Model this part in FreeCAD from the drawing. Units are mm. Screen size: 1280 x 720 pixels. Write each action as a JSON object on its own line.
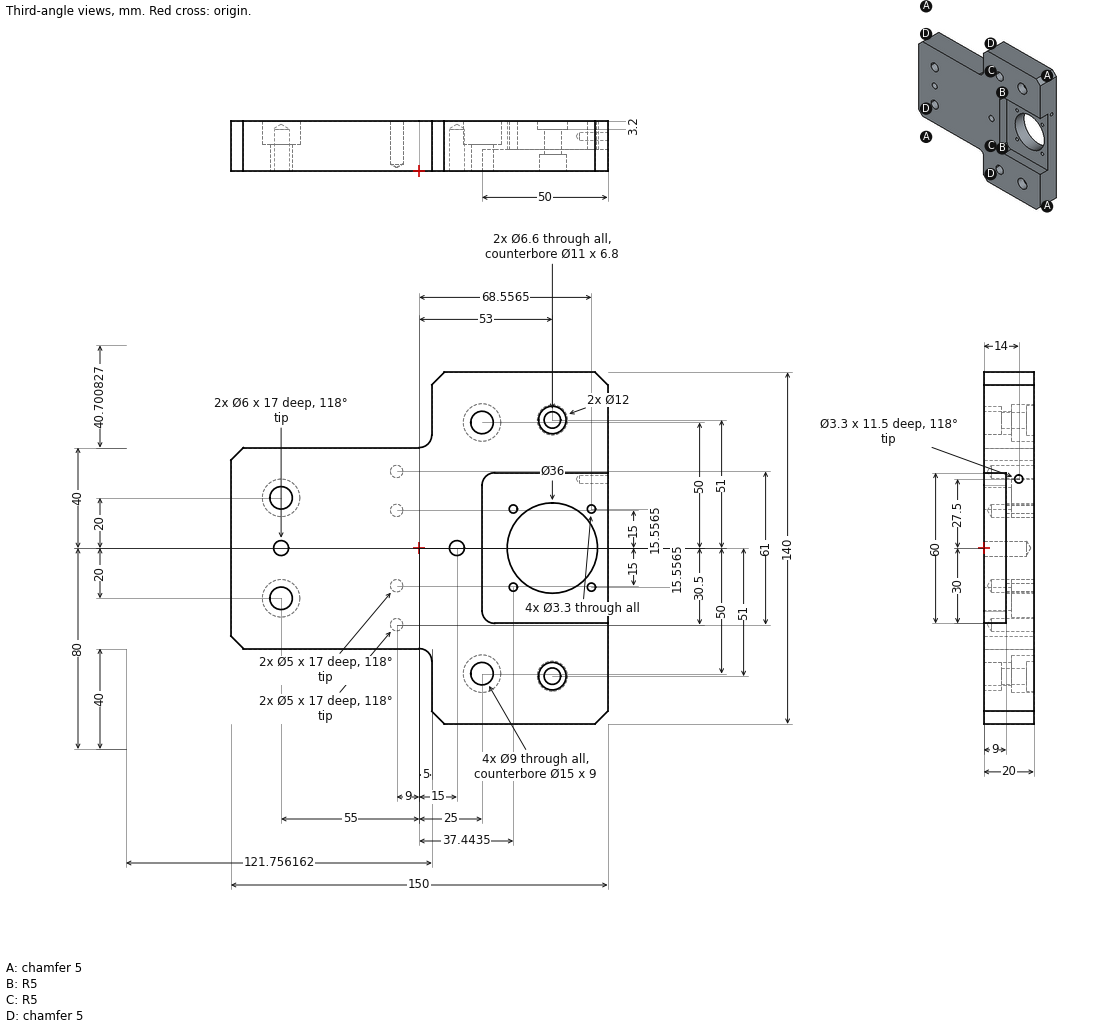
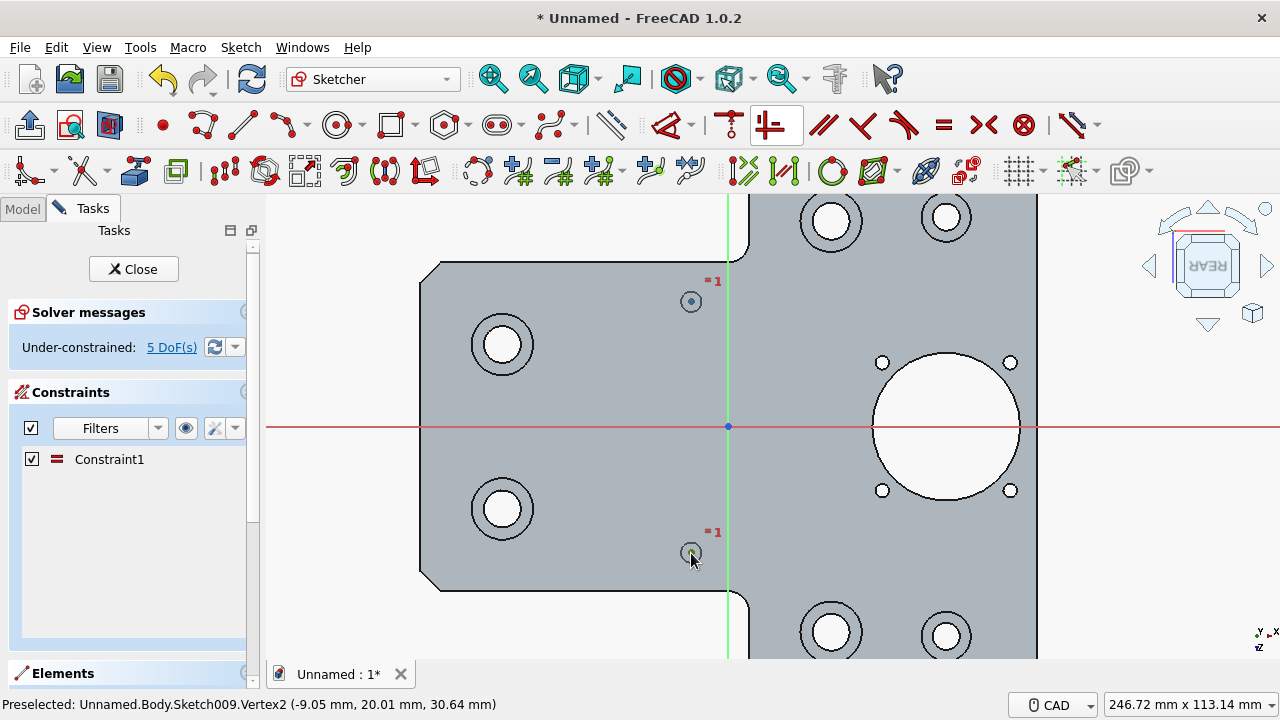
{"action": "key", "text": "v"}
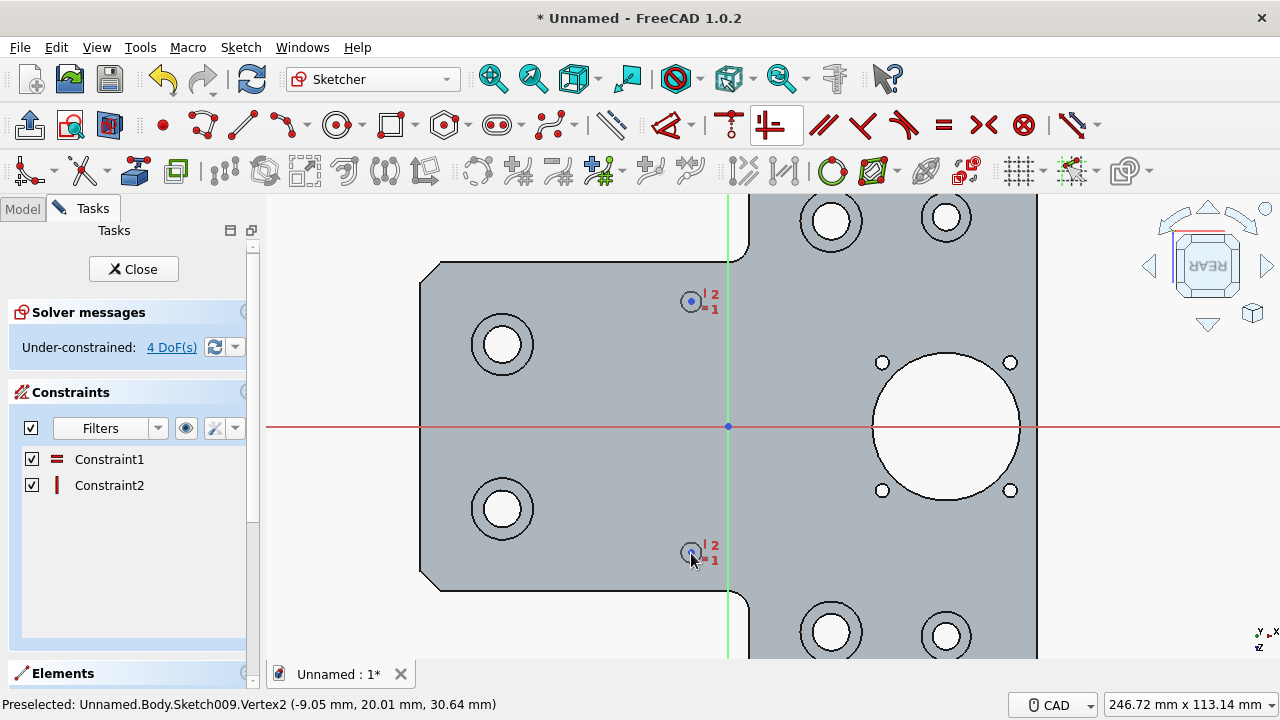
{"action": "left_click", "coordinate": [666, 126]}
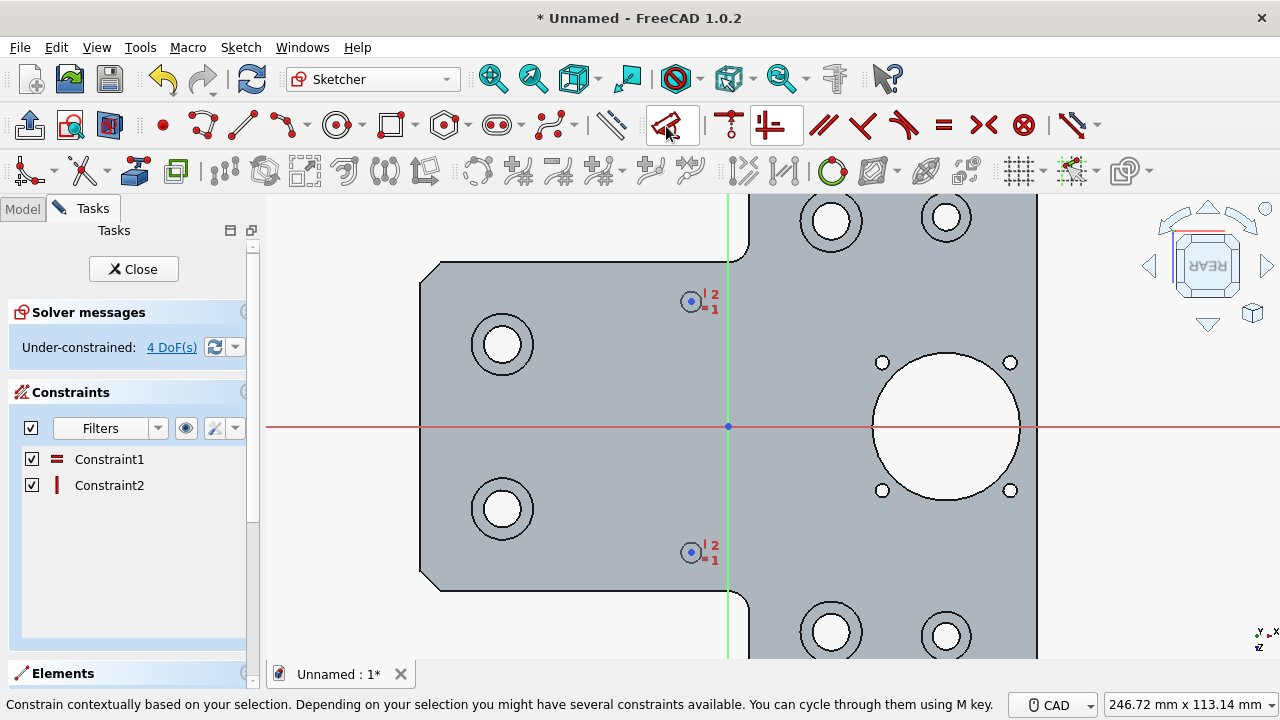
{"action": "scroll", "coordinate": [698, 295], "scroll_direction": "up", "scroll_amount": 4}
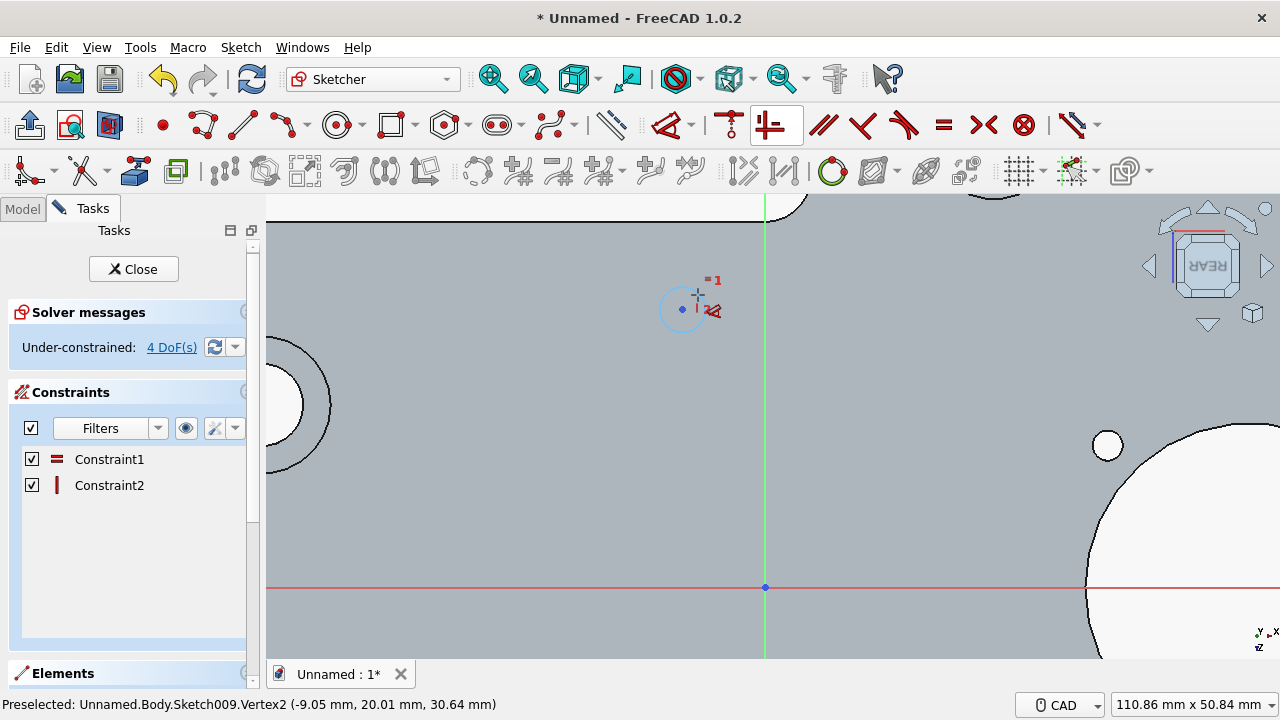
{"action": "left_click", "coordinate": [699, 294]}
{"action": "left_click", "coordinate": [722, 272]}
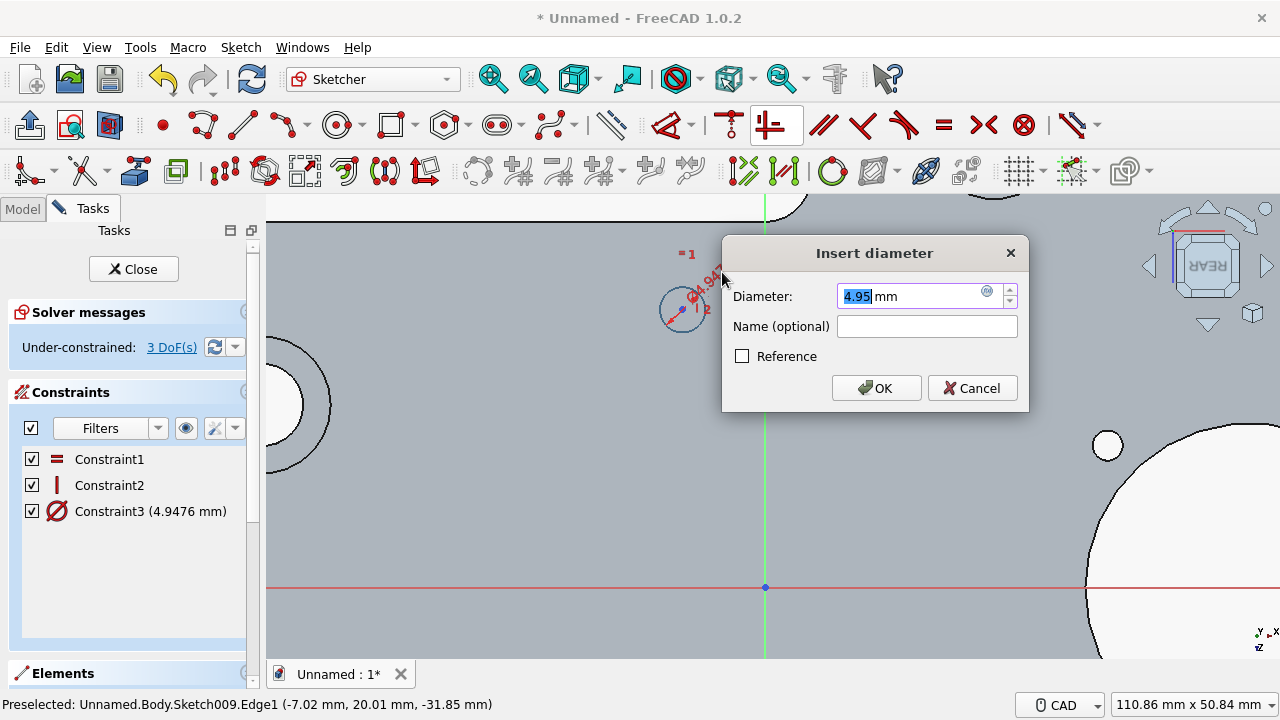
{"action": "type", "text": "5"}
{"action": "key", "text": "Return"}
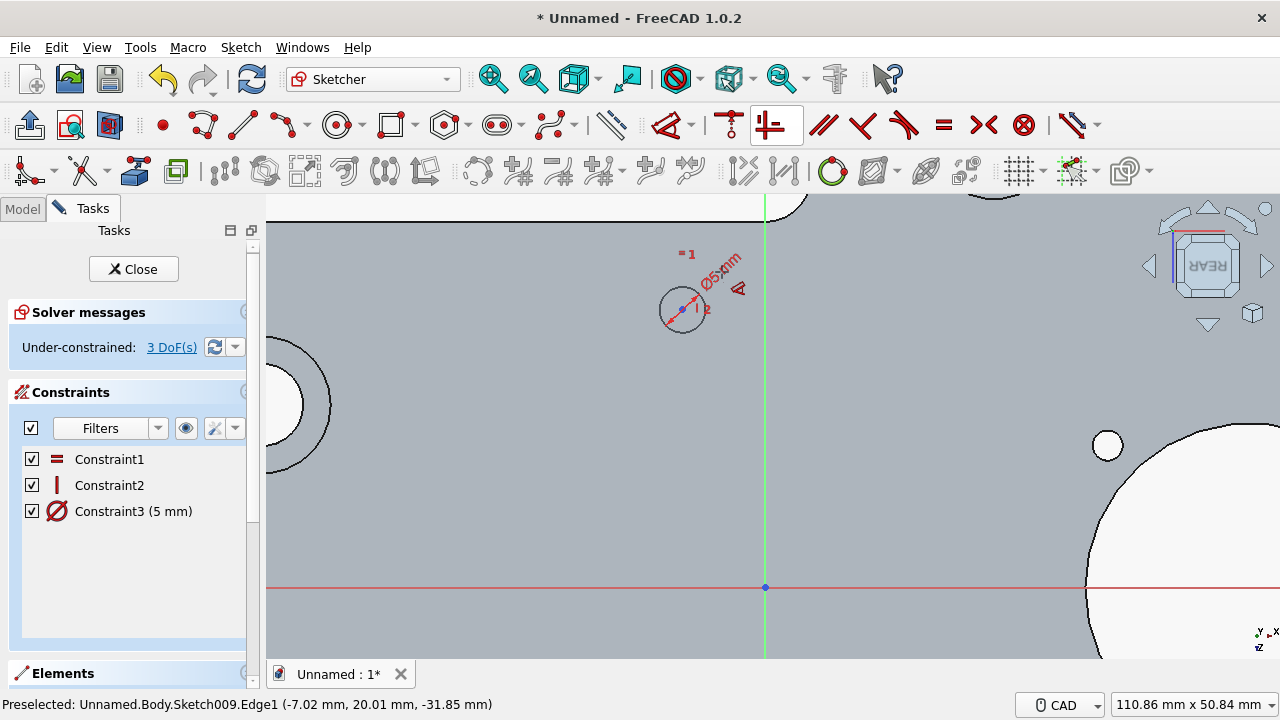
{"action": "left_click", "coordinate": [683, 310]}
{"action": "left_click", "coordinate": [724, 622]}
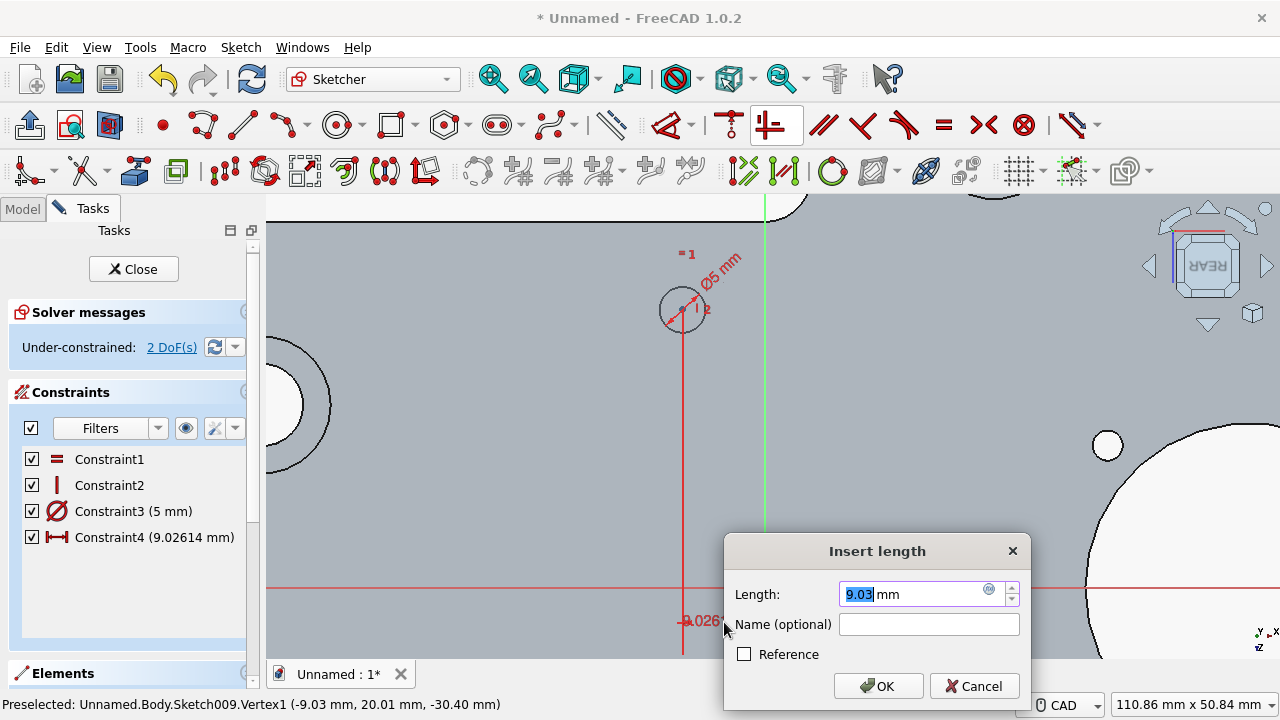
{"action": "type", "text": "9"}
{"action": "key", "text": "Return"}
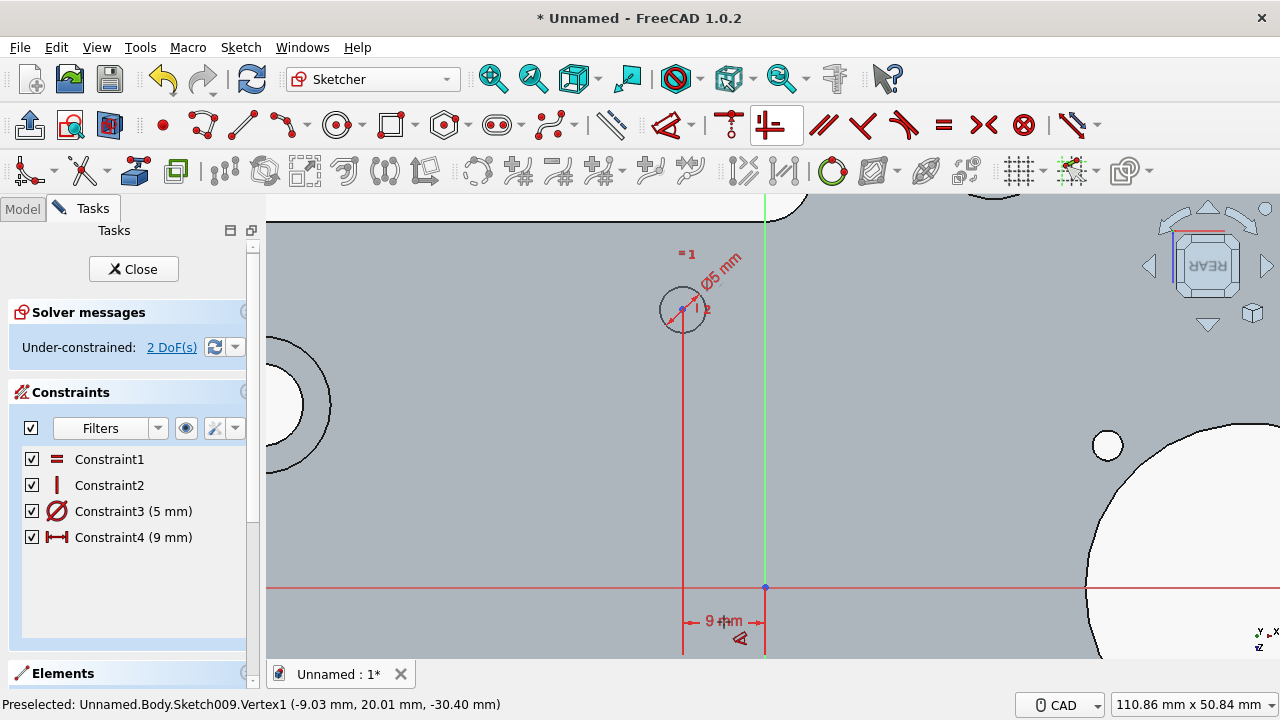
{"action": "left_click", "coordinate": [683, 310]}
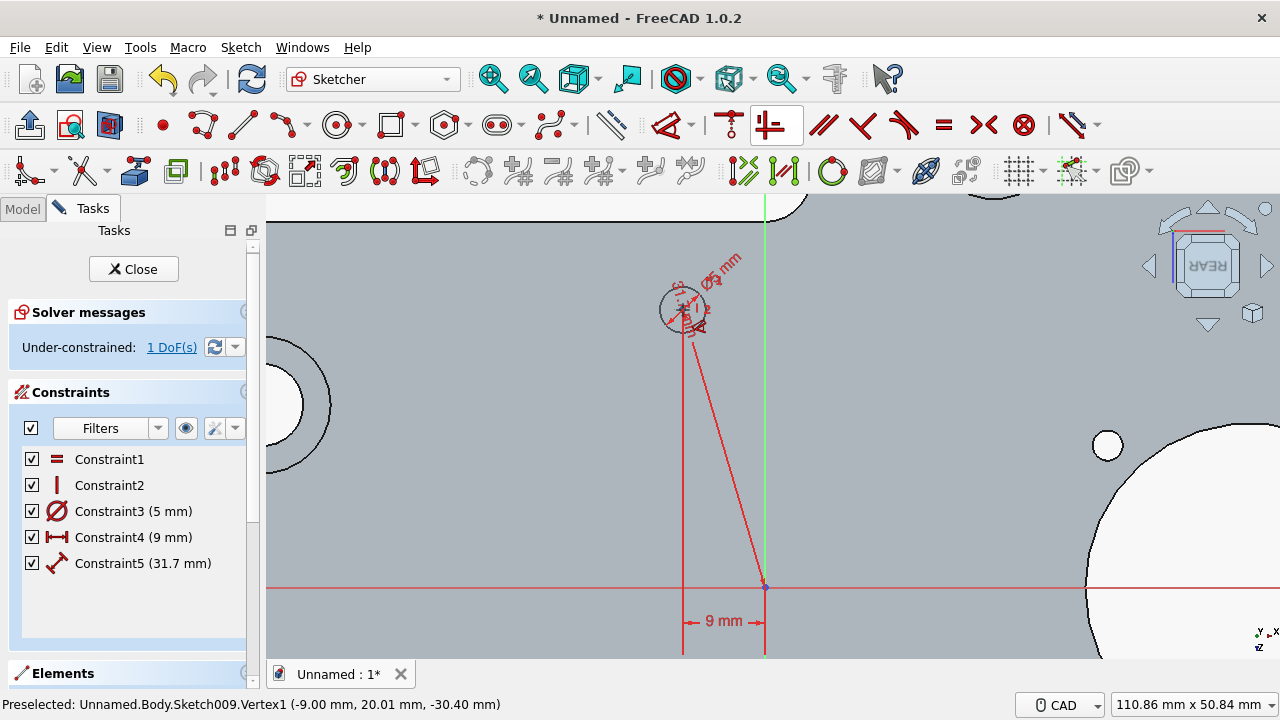
{"action": "scroll", "coordinate": [698, 295], "scroll_direction": "down", "scroll_amount": 4}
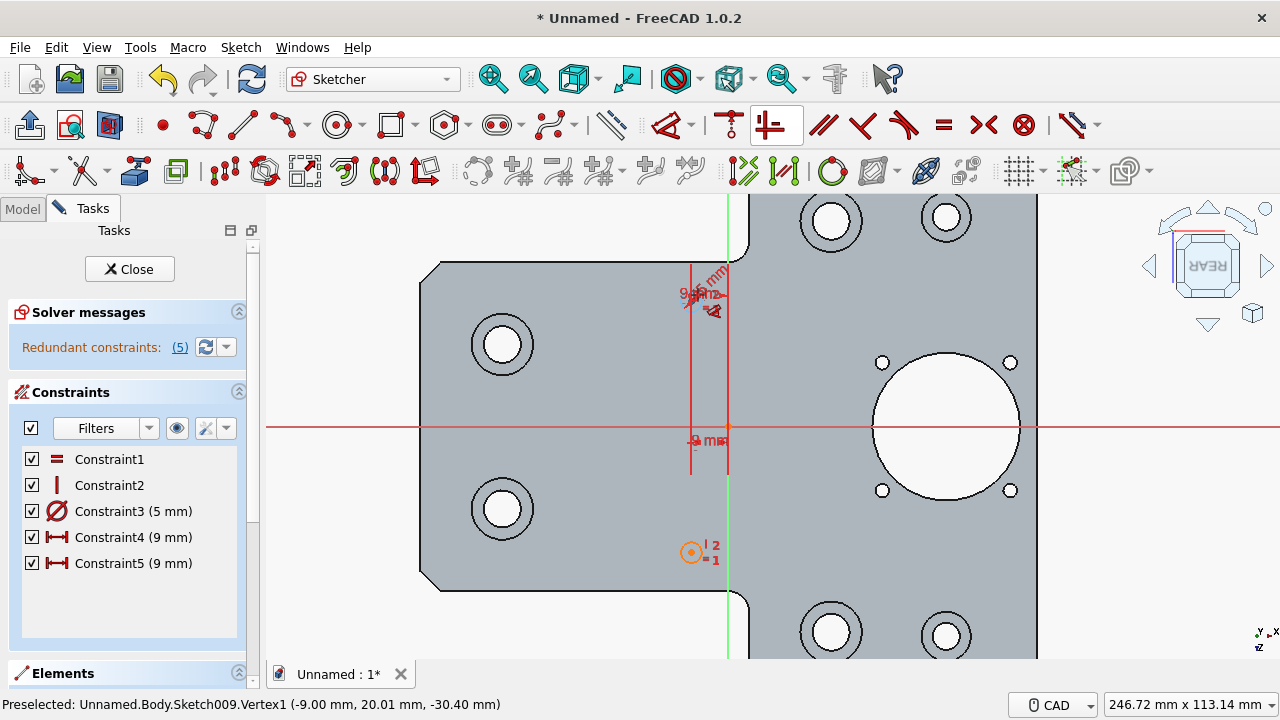
{"action": "left_click", "coordinate": [691, 553]}
{"action": "left_click", "coordinate": [657, 370]}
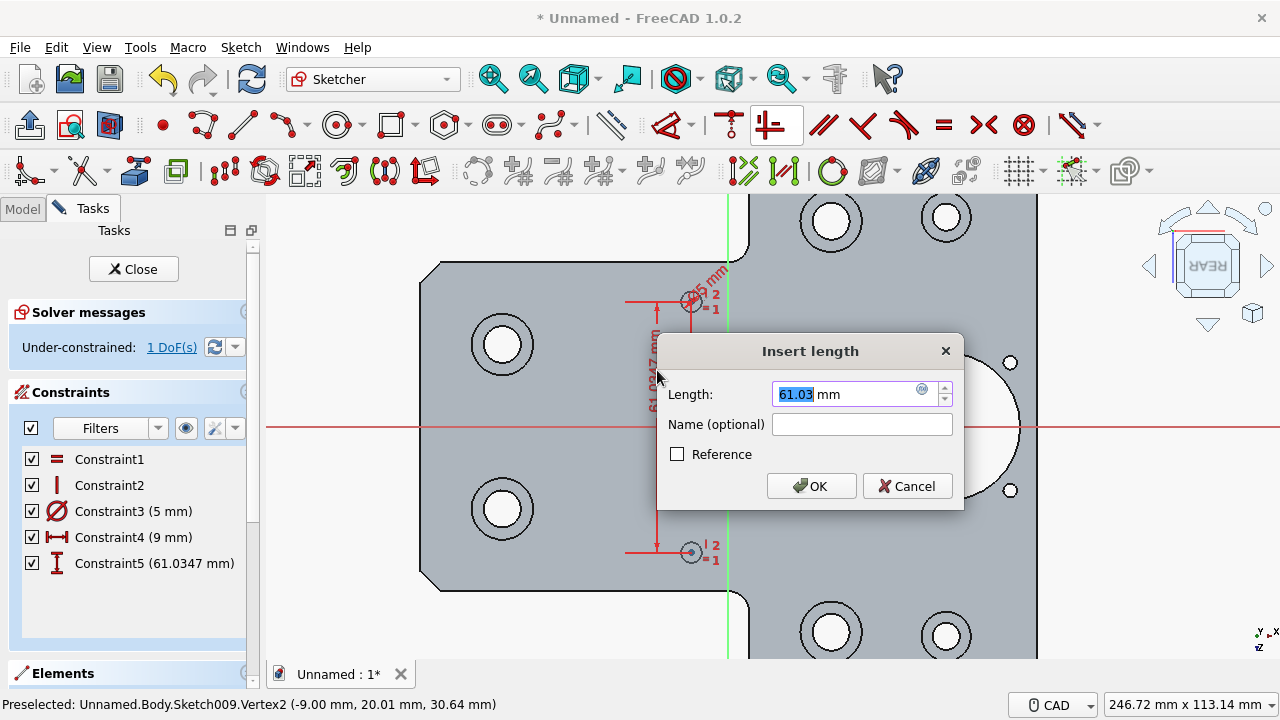
{"action": "type", "text": "61"}
{"action": "key", "text": "Return"}